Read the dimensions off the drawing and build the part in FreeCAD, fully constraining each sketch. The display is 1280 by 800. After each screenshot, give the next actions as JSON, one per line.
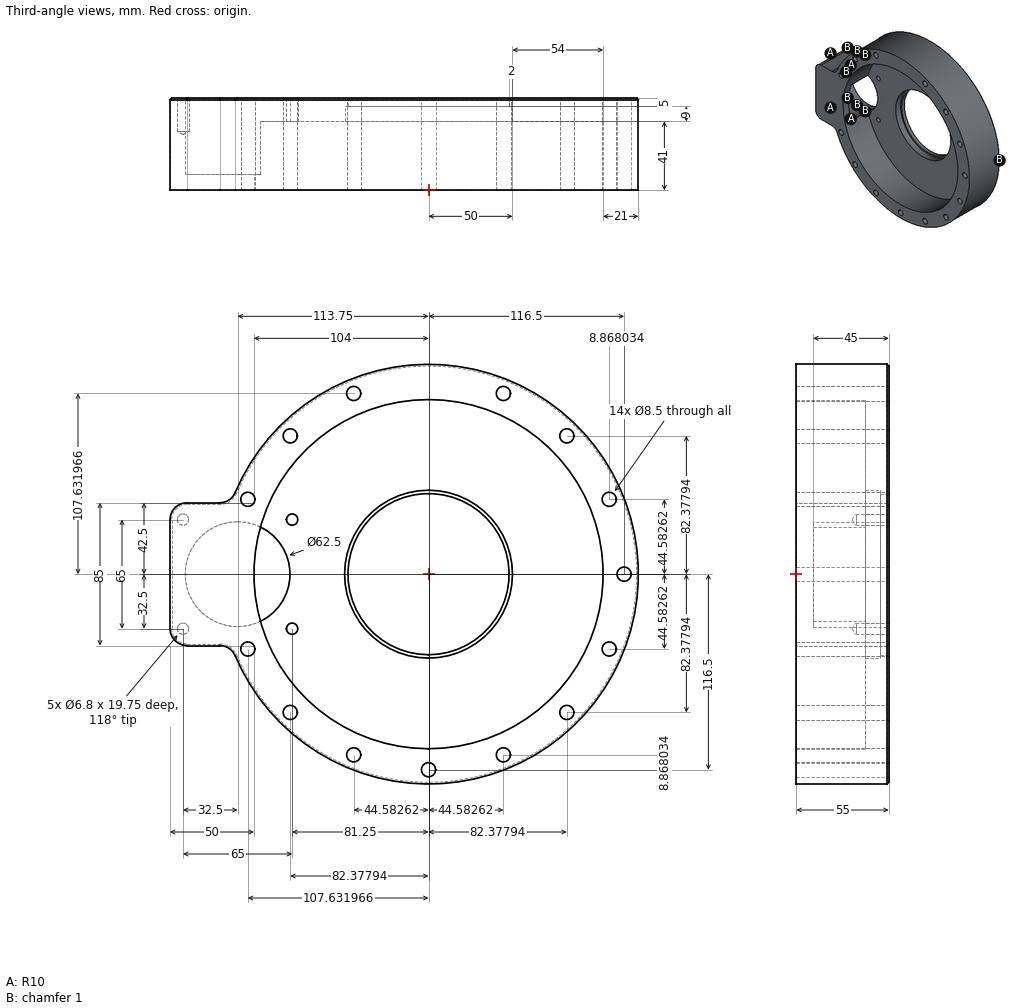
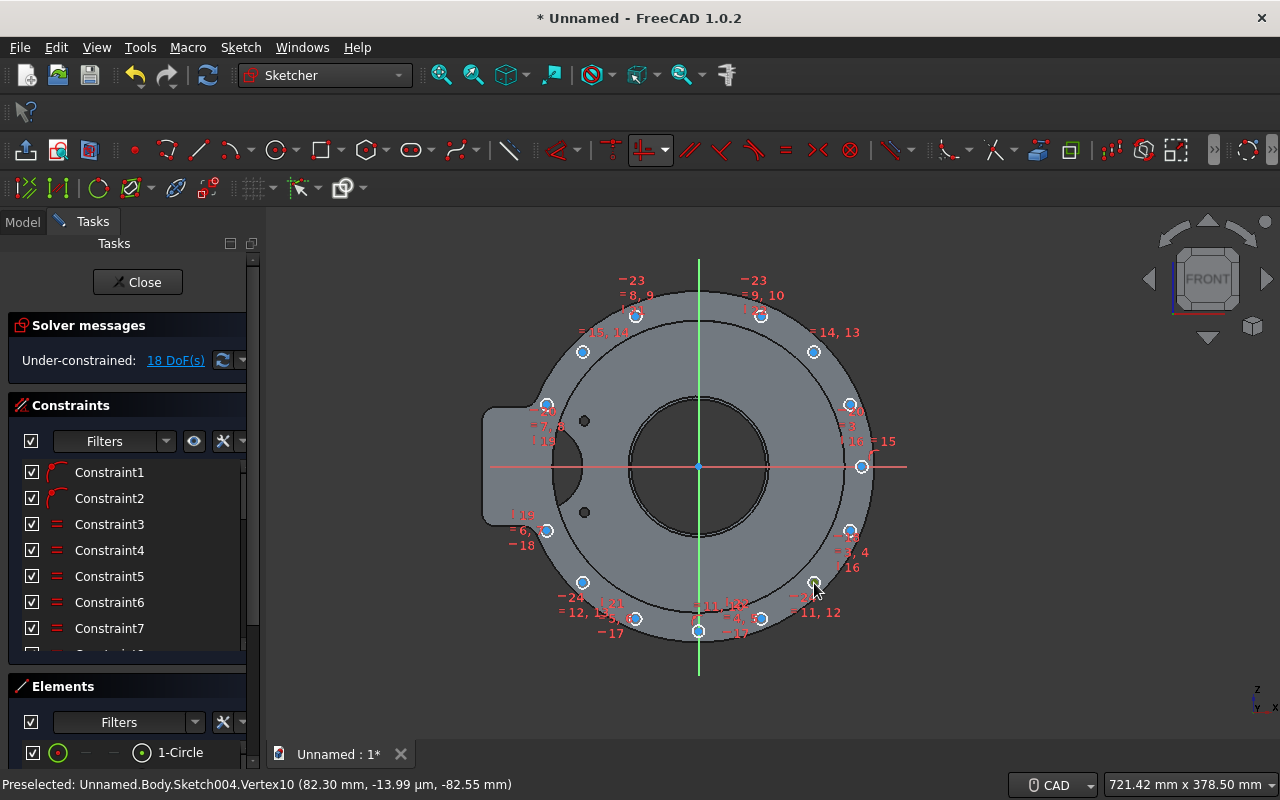
{"action": "left_click", "coordinate": [814, 352]}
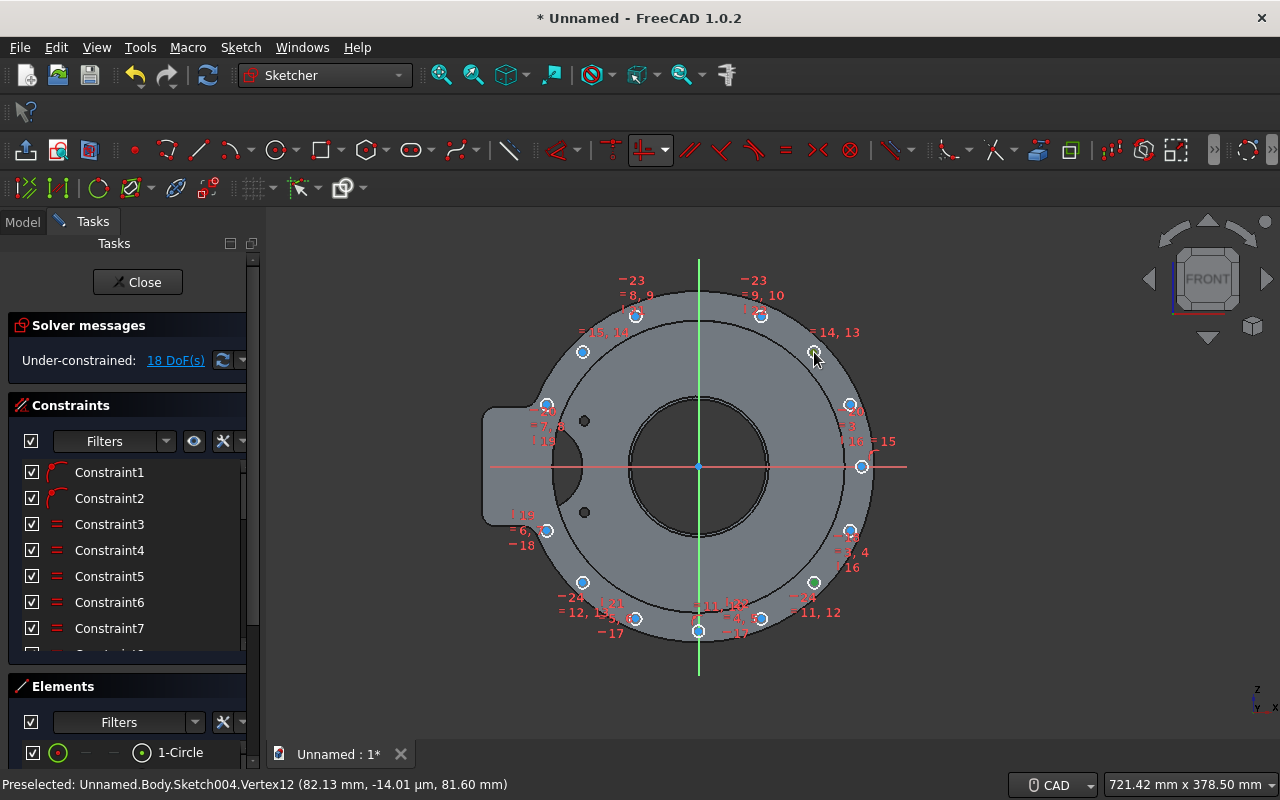
{"action": "key", "text": "v"}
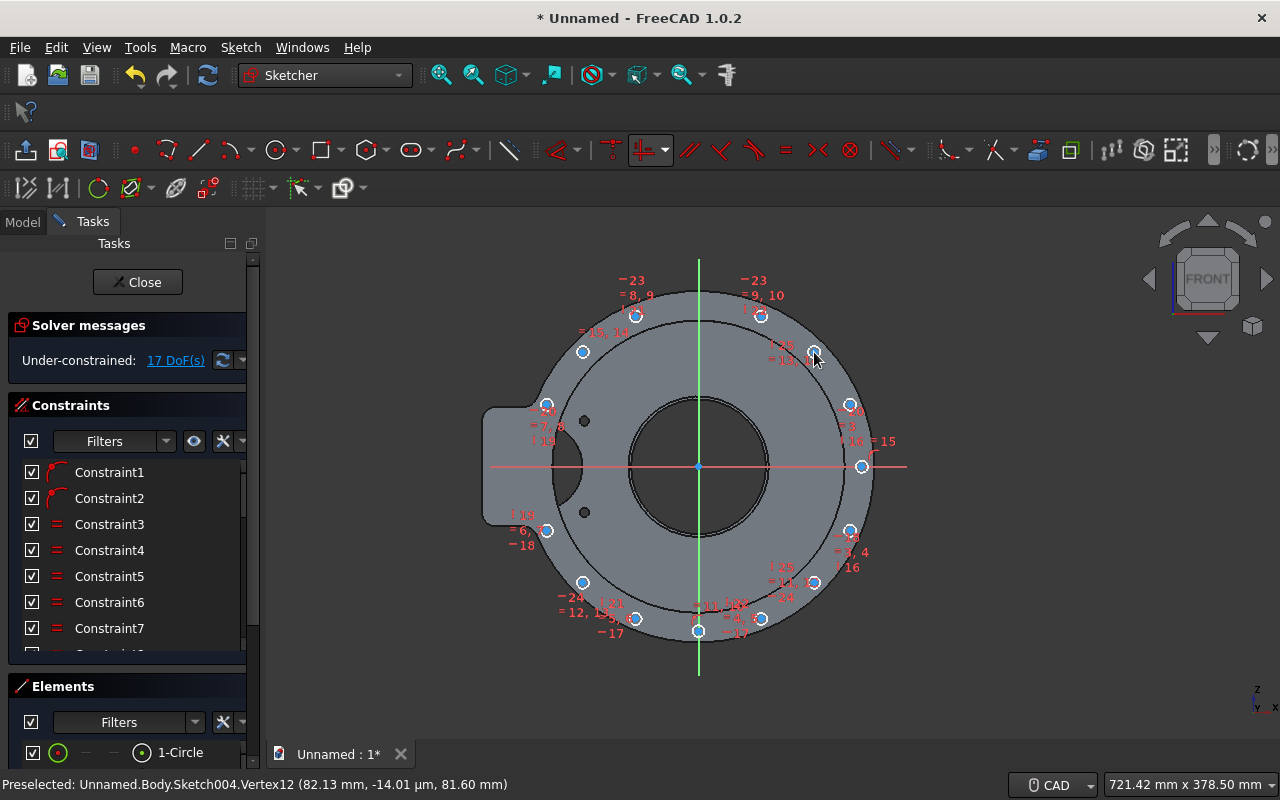
{"action": "left_click", "coordinate": [583, 583]}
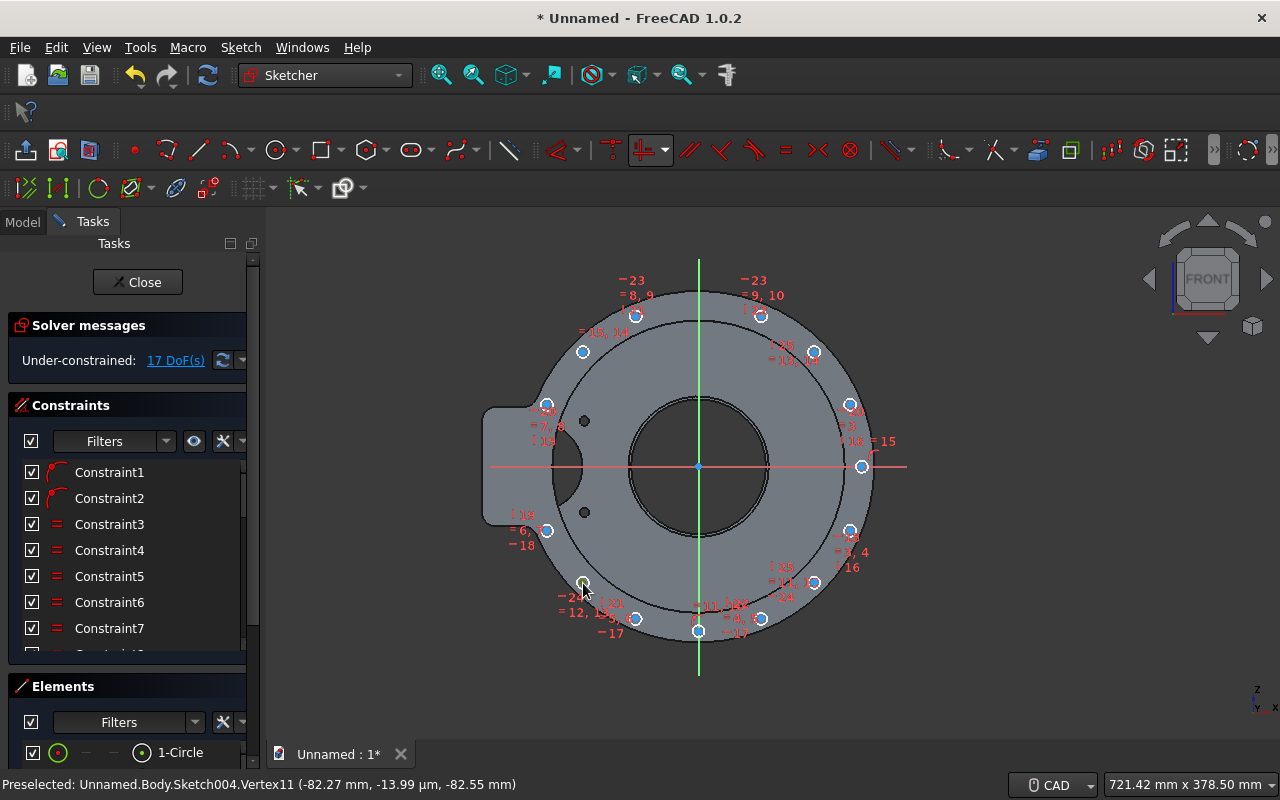
{"action": "left_click", "coordinate": [583, 352]}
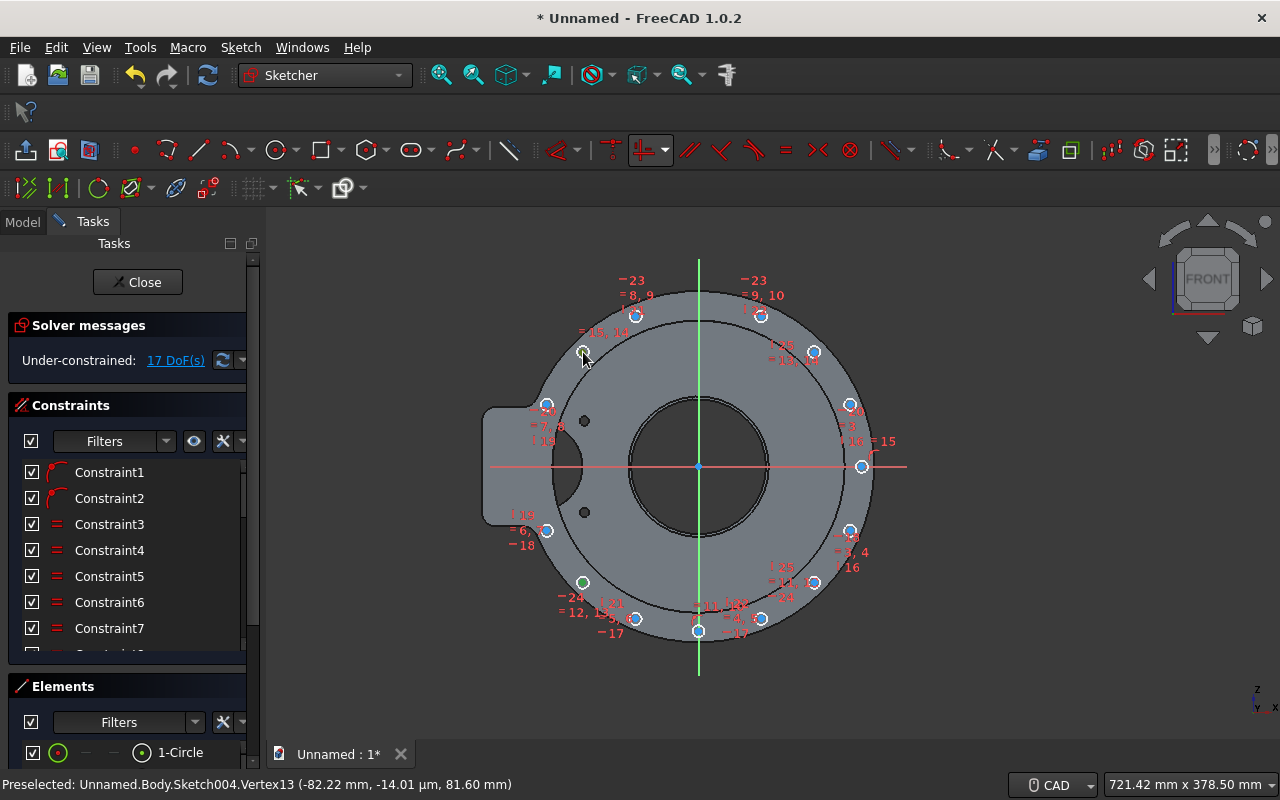
{"action": "left_click", "coordinate": [668, 150]}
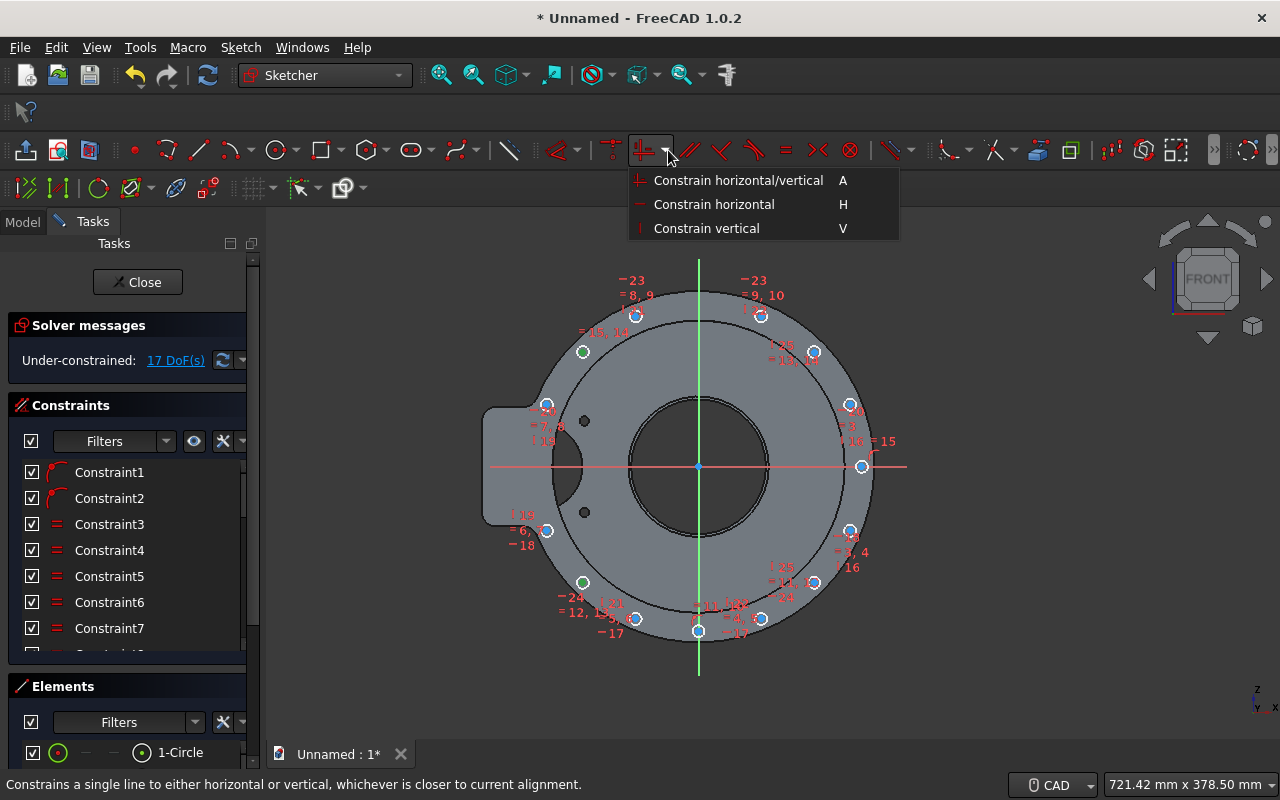
{"action": "left_click", "coordinate": [764, 228]}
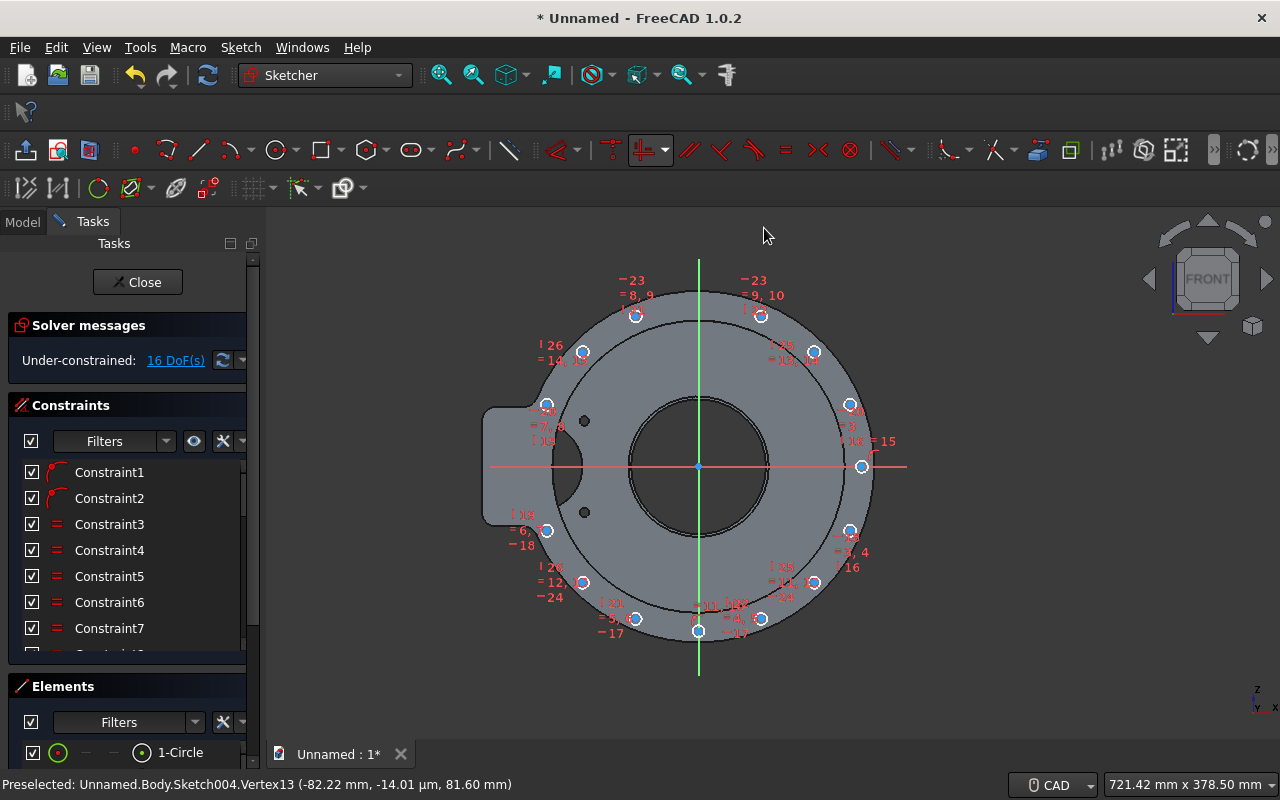
{"action": "scroll", "coordinate": [814, 352], "scroll_direction": "up", "scroll_amount": 4}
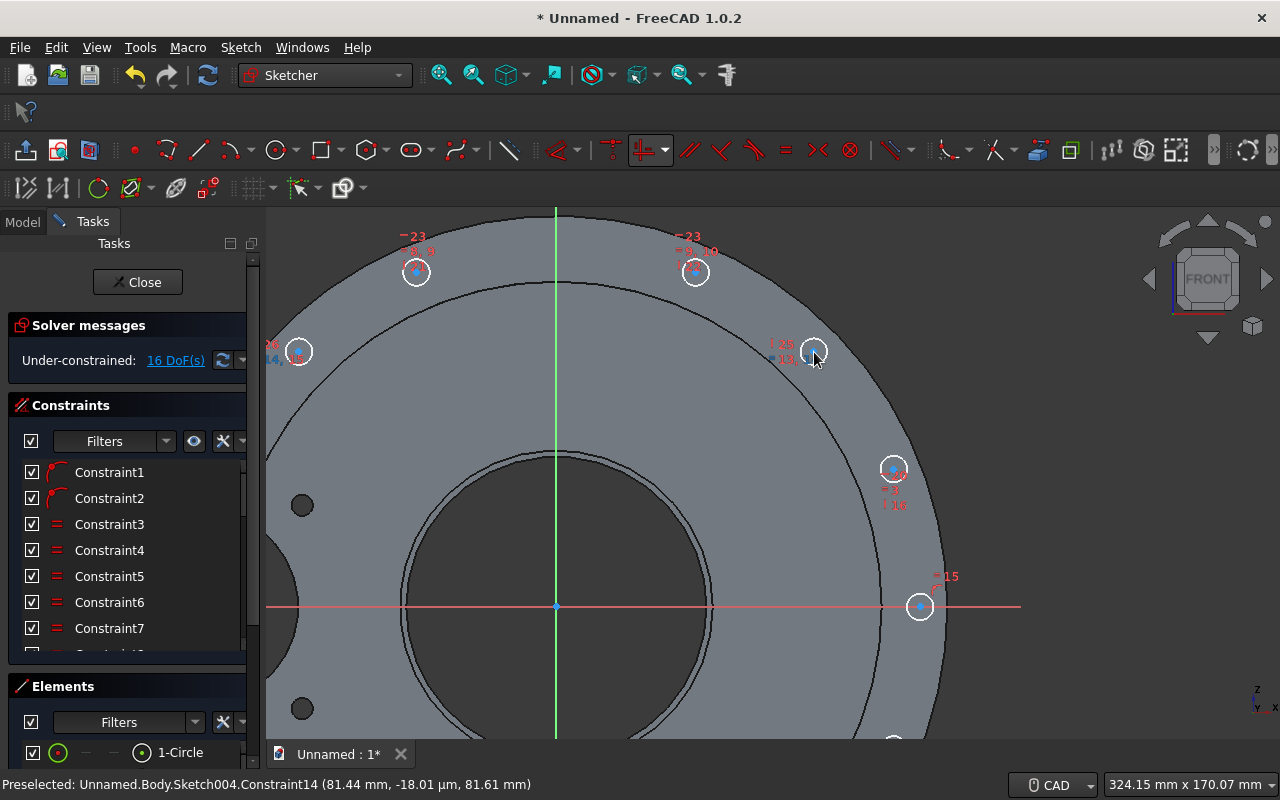
{"action": "scroll", "coordinate": [814, 352], "scroll_direction": "up", "scroll_amount": 4}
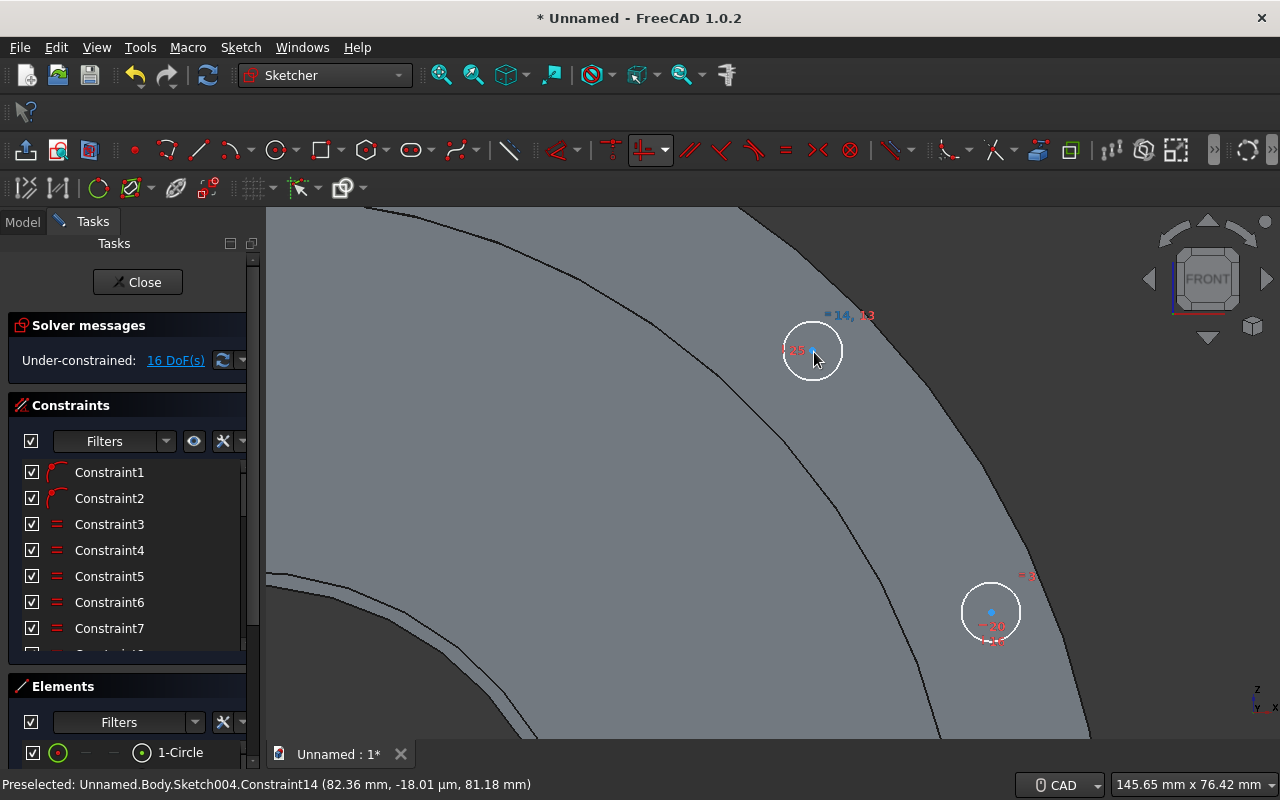
{"action": "left_click", "coordinate": [813, 351]}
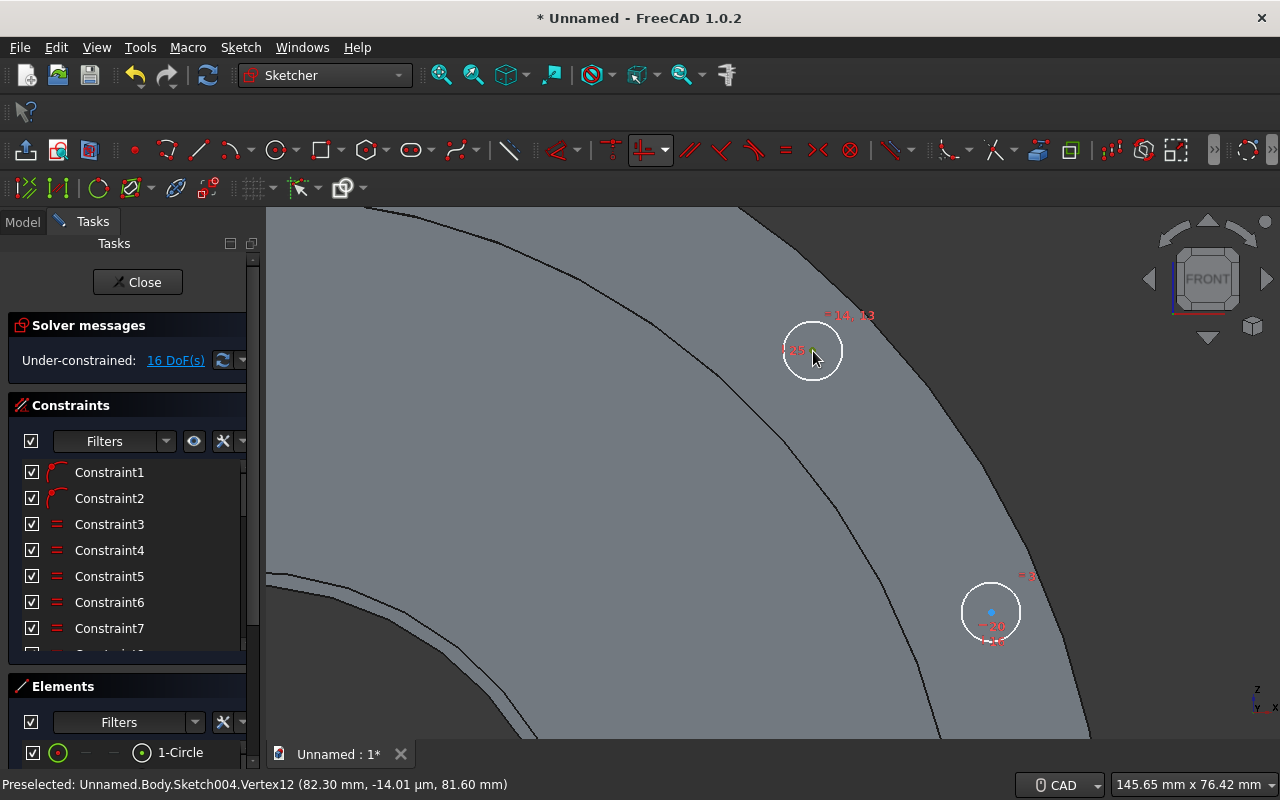
{"action": "scroll", "coordinate": [814, 352], "scroll_direction": "down", "scroll_amount": 8}